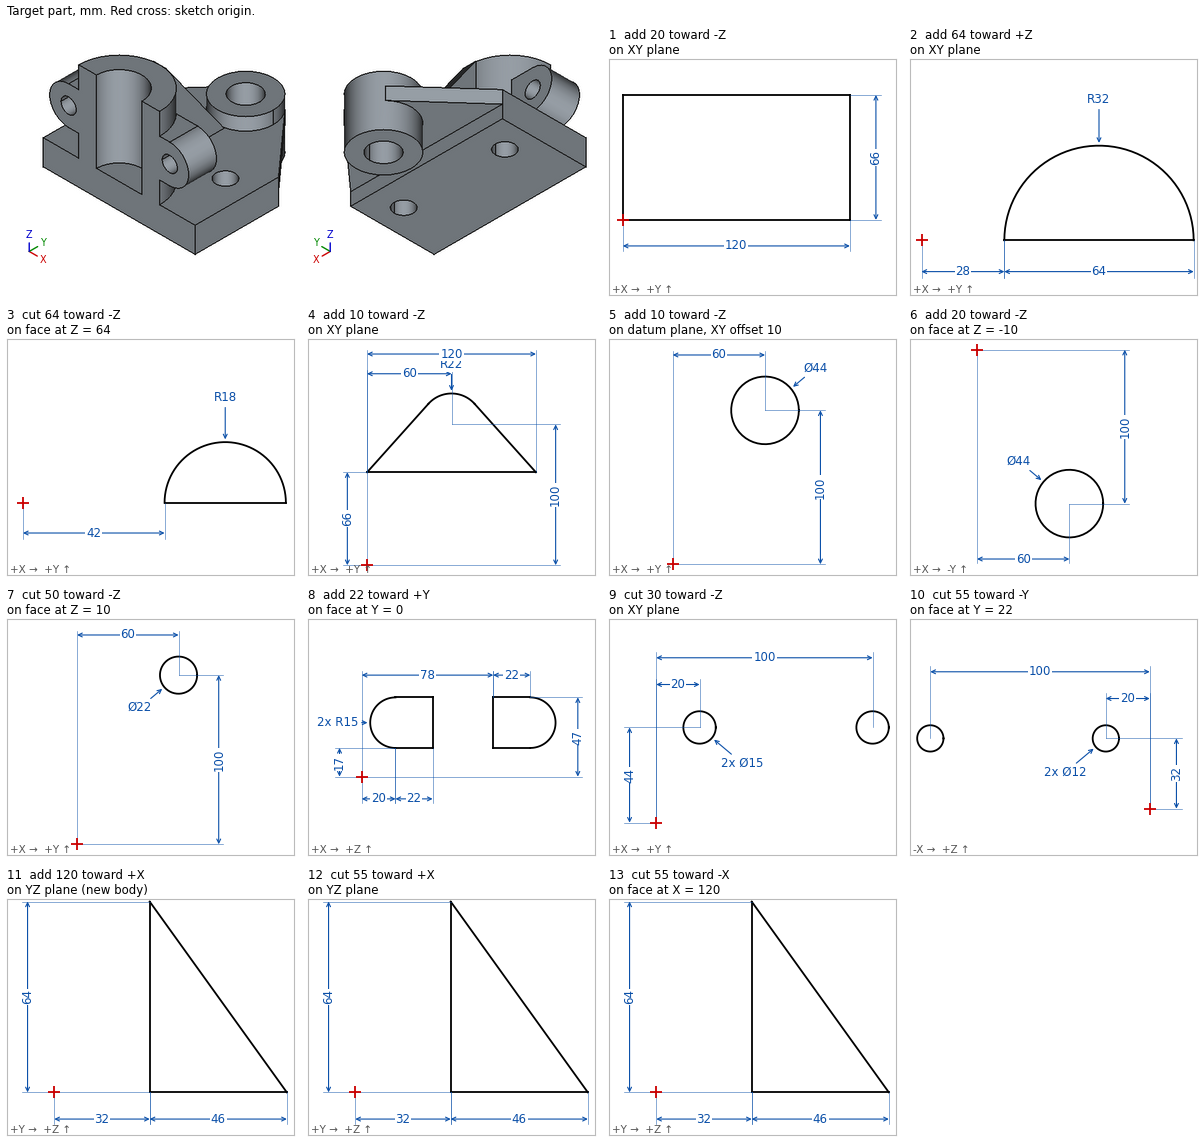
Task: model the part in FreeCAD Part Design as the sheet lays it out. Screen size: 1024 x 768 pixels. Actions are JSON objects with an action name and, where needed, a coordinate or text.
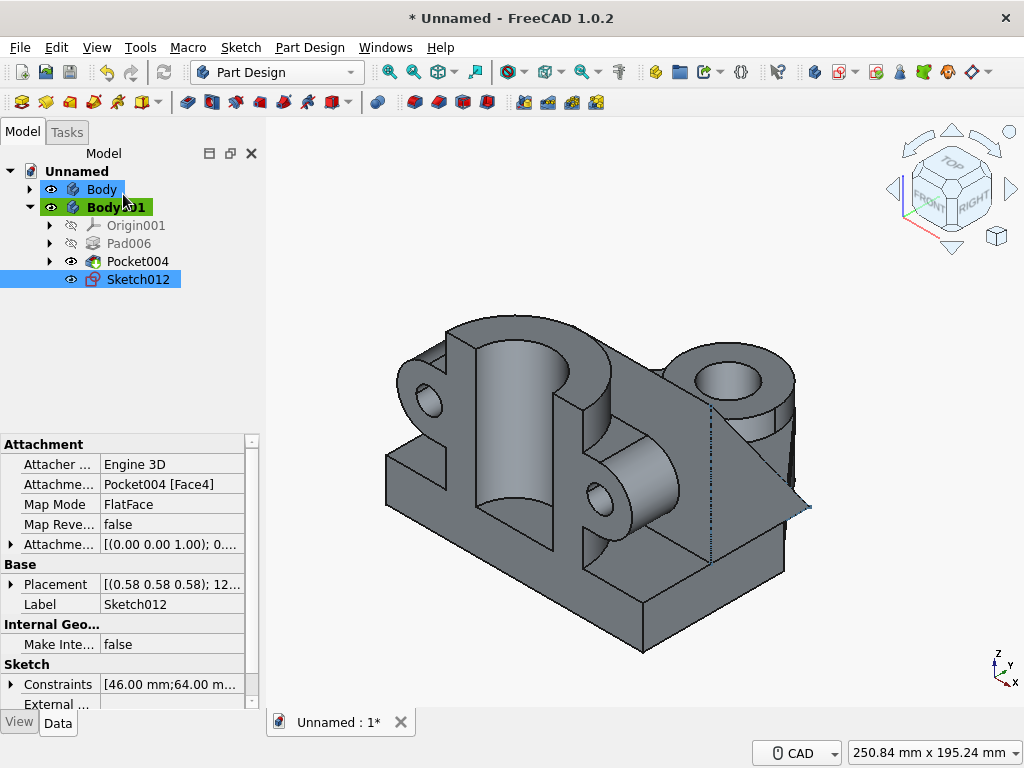
{"action": "left_click", "coordinate": [188, 102]}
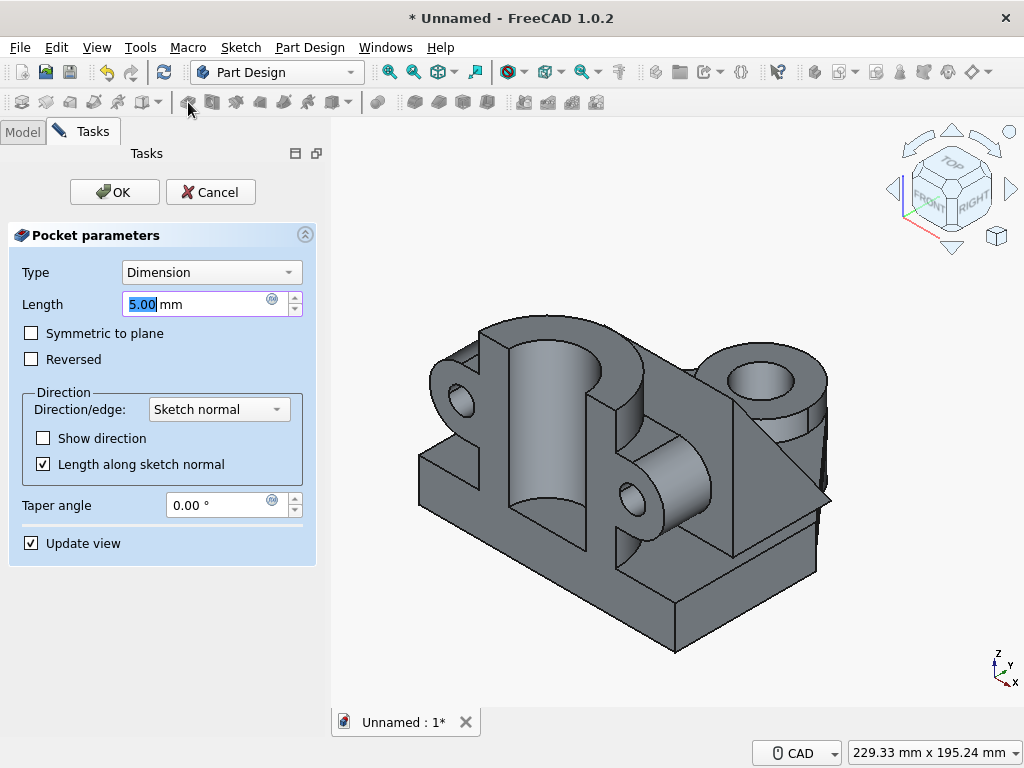
{"action": "type", "text": "55"}
{"action": "key", "text": "Tab"}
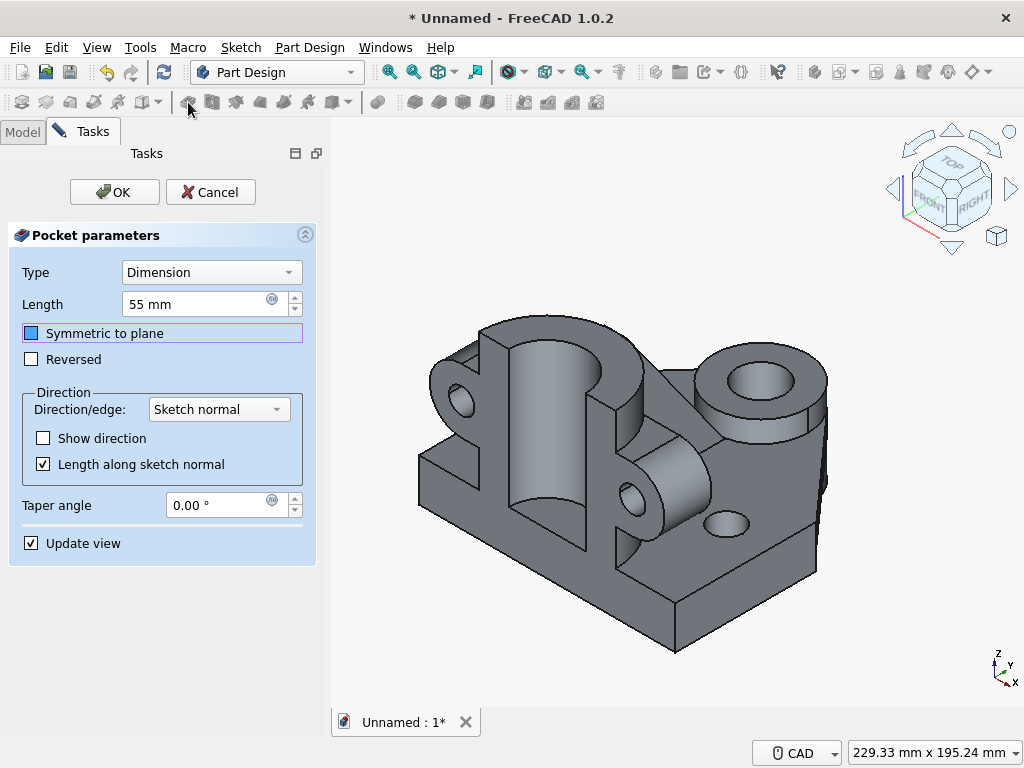
{"action": "left_click", "coordinate": [115, 192]}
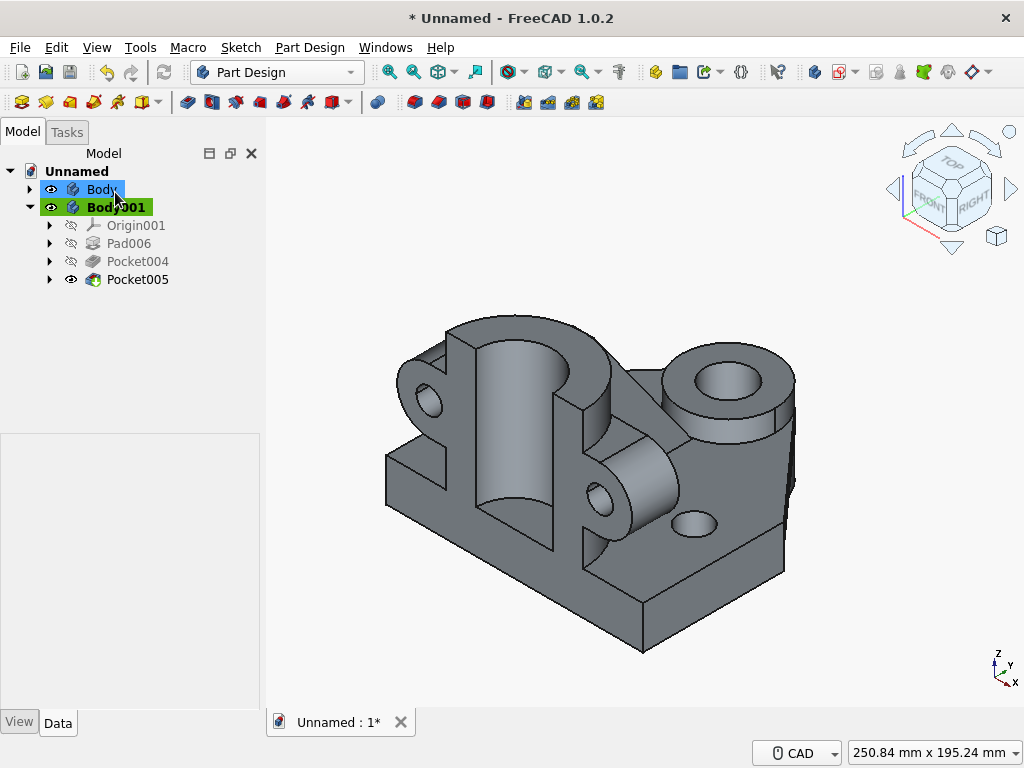
{"action": "left_click", "coordinate": [390, 72]}